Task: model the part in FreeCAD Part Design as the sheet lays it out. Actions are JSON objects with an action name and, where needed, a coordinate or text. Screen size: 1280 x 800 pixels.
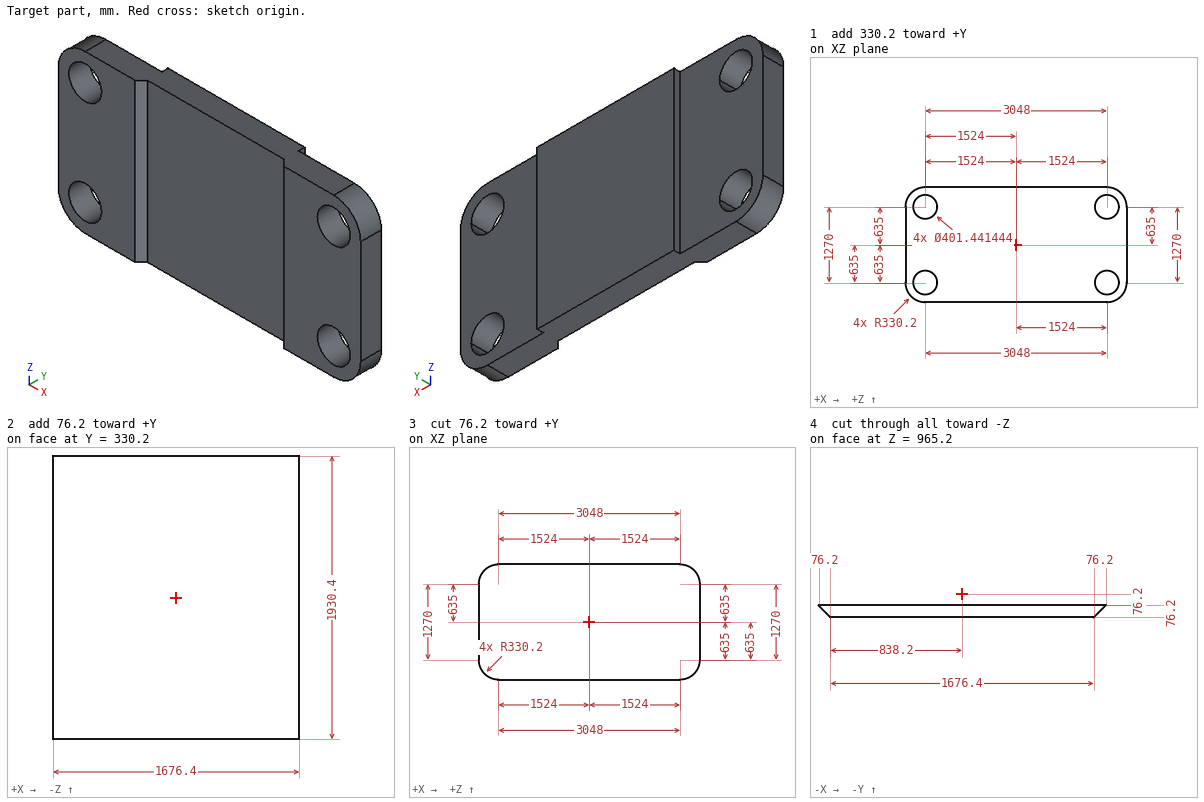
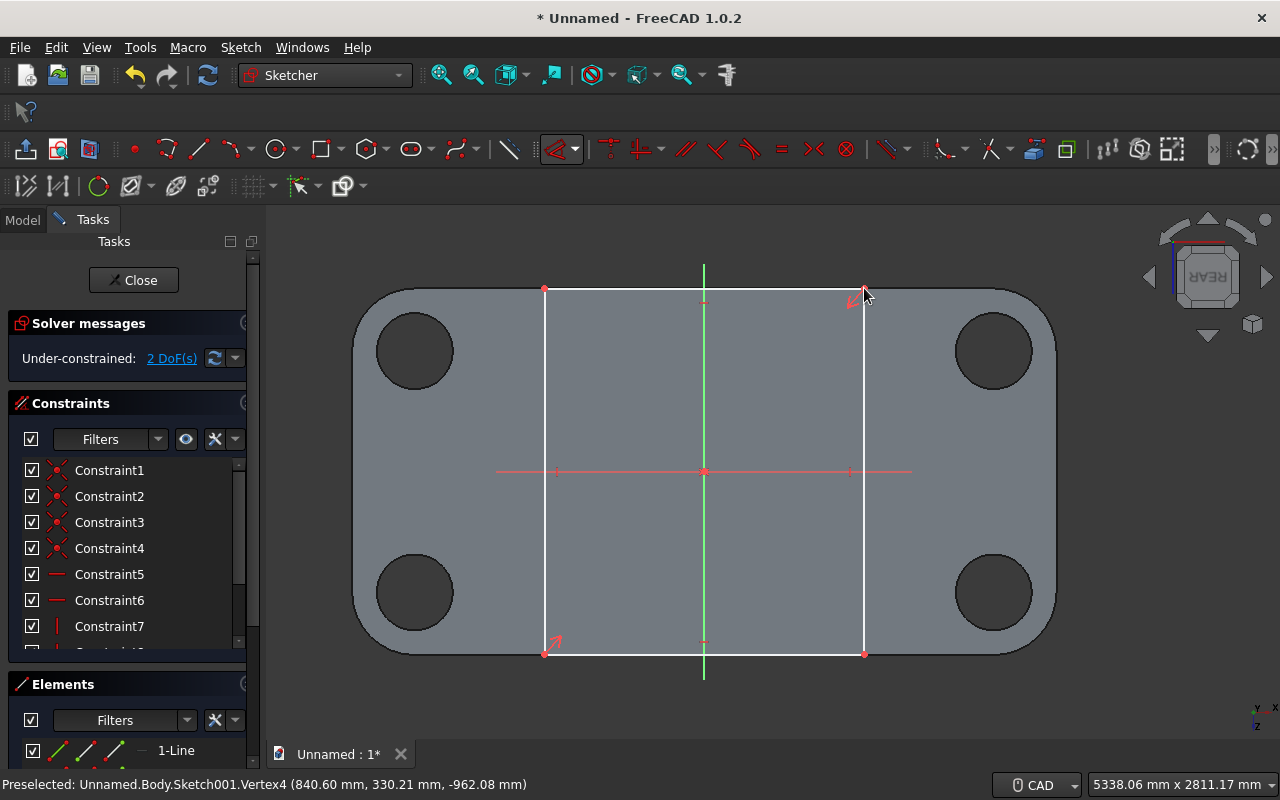
{"action": "left_click", "coordinate": [640, 655]}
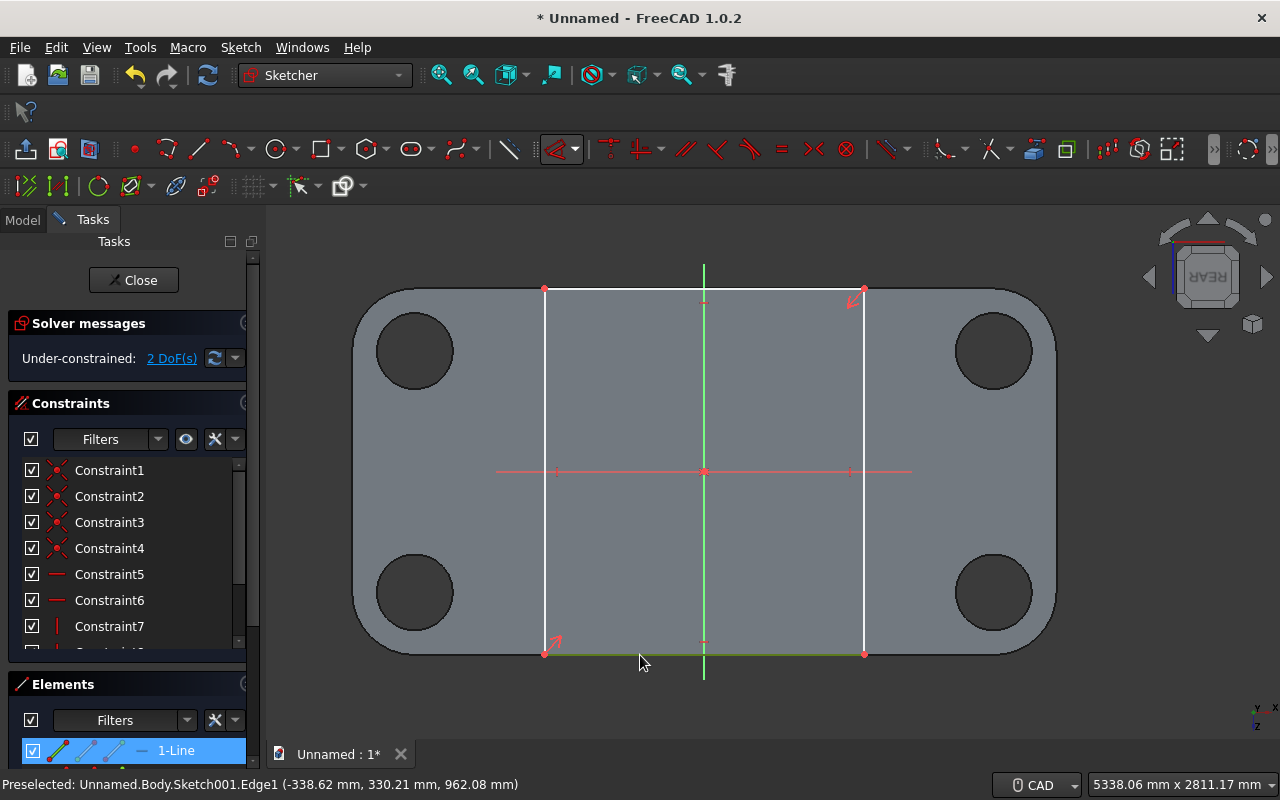
{"action": "key", "text": "l"}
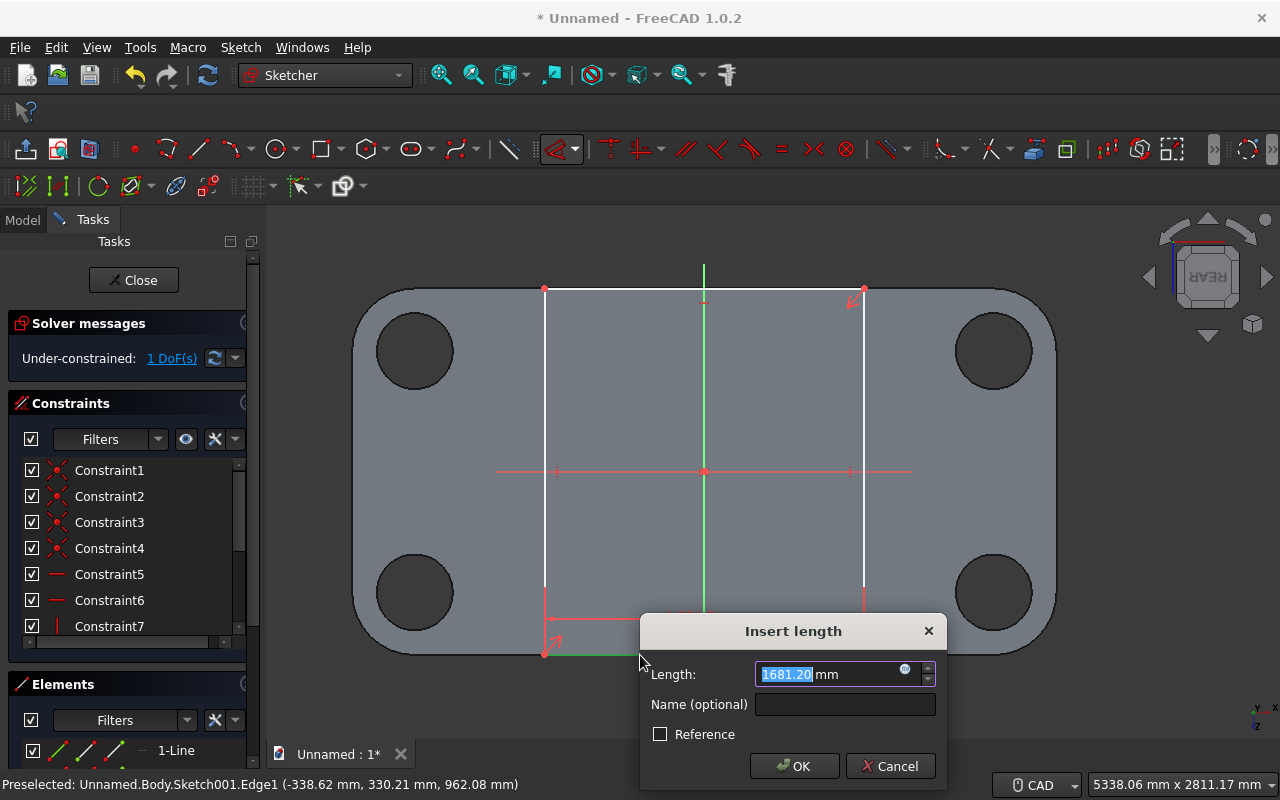
{"action": "type", "text": "1676.4"}
{"action": "key", "text": "Return"}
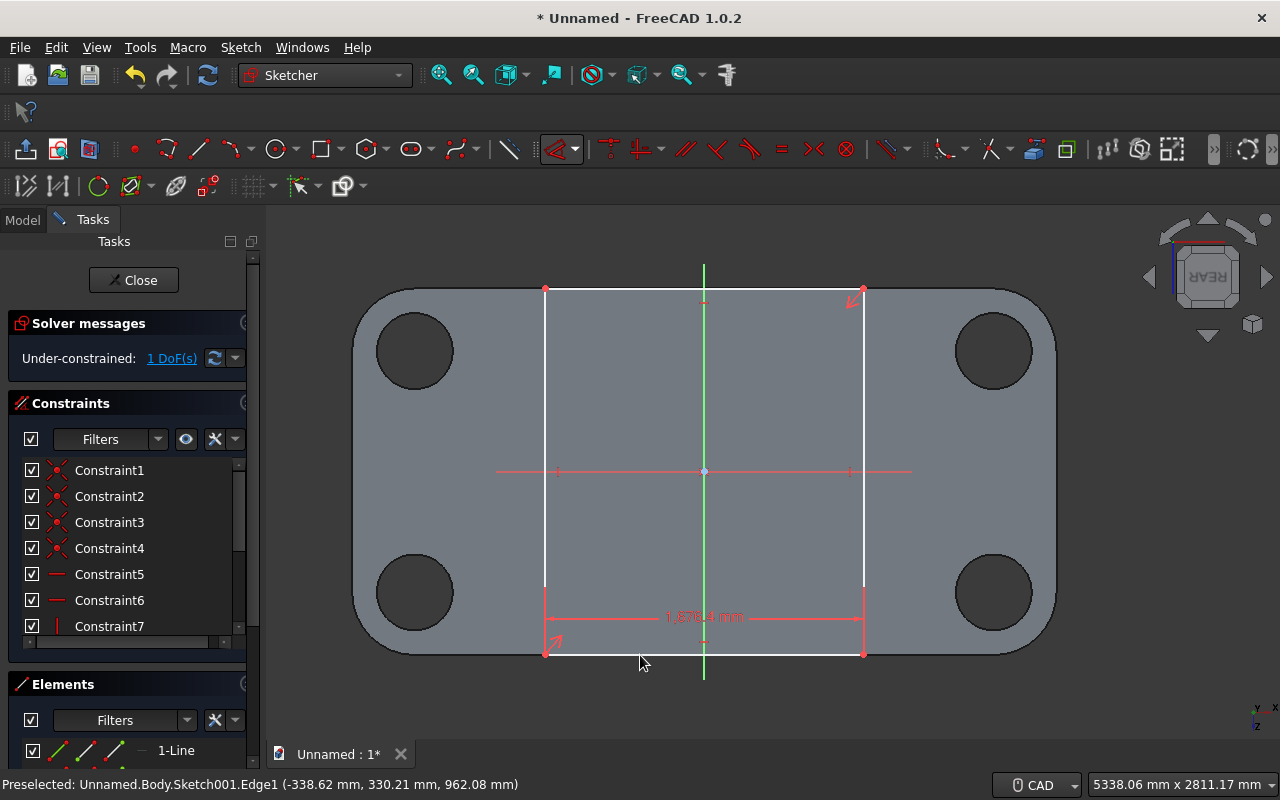
{"action": "left_click", "coordinate": [864, 545]}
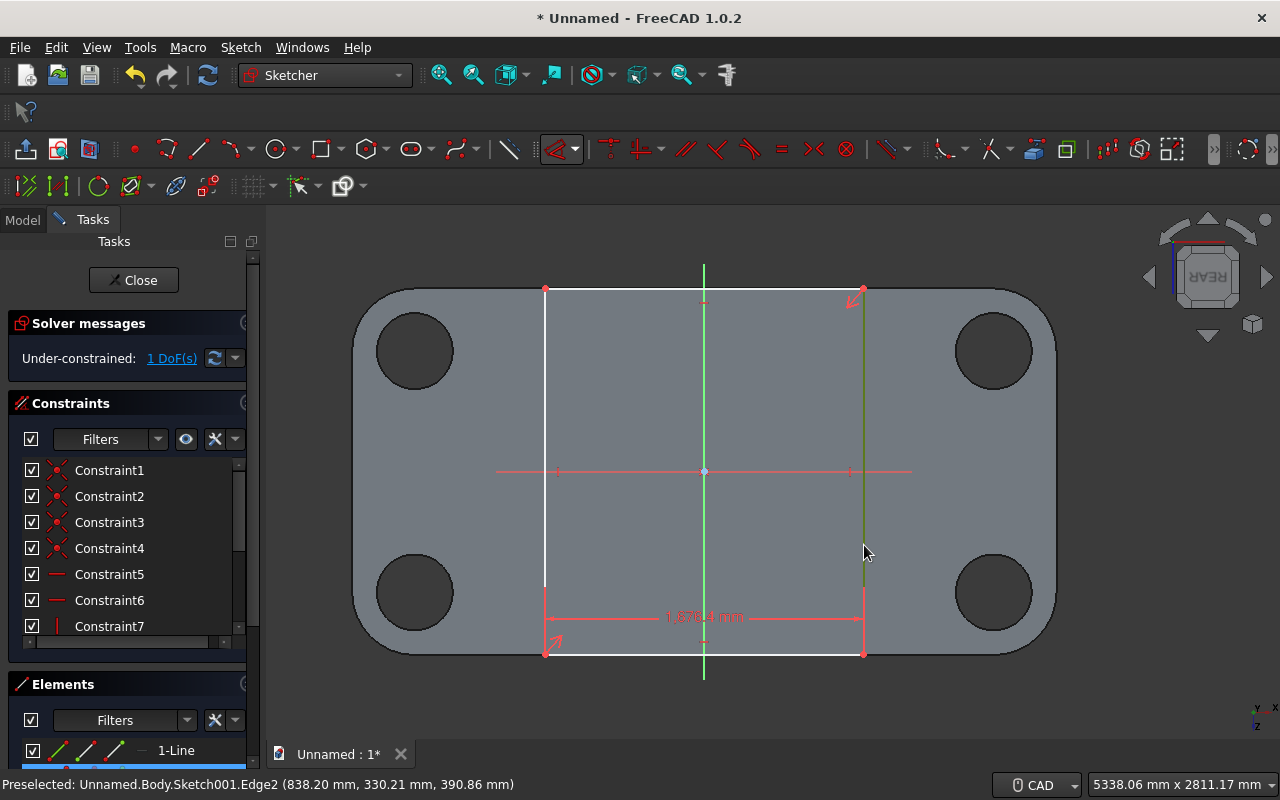
{"action": "key", "text": "i"}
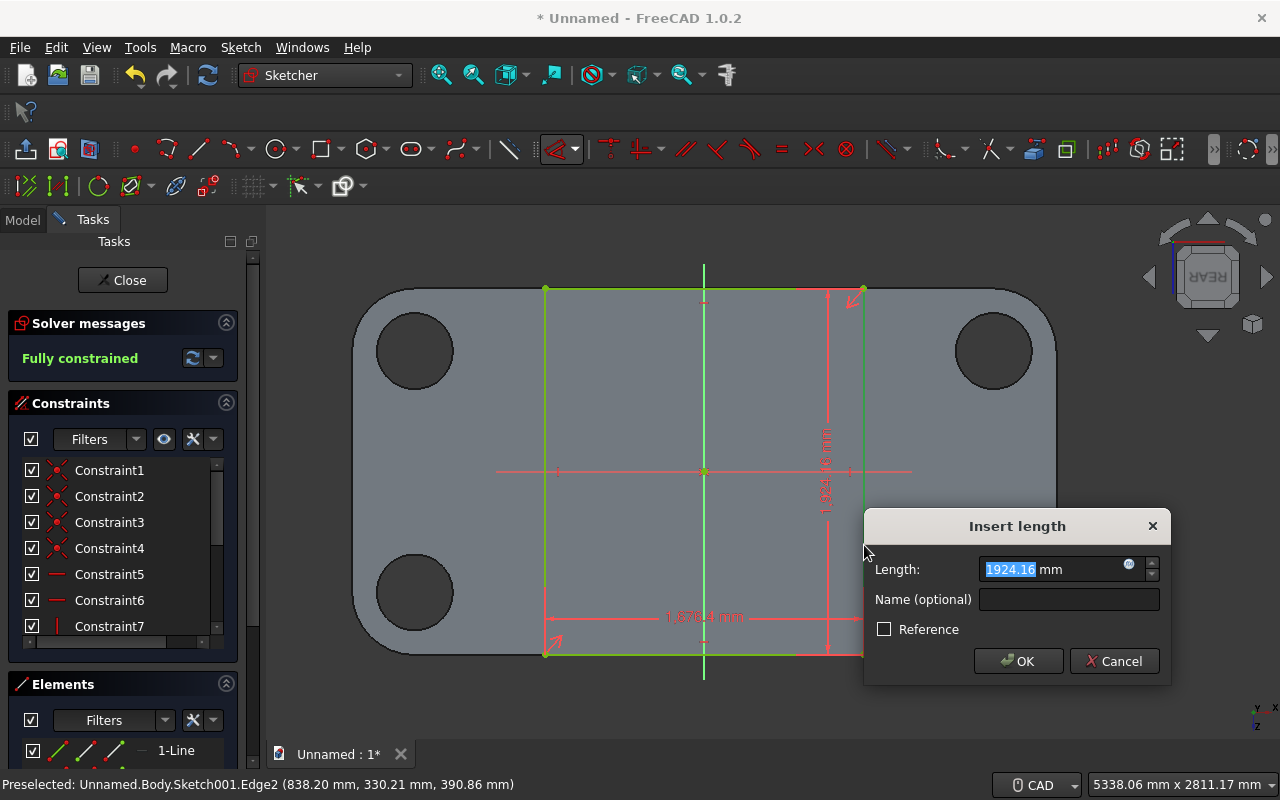
{"action": "type", "text": "1930.4"}
{"action": "key", "text": "Return"}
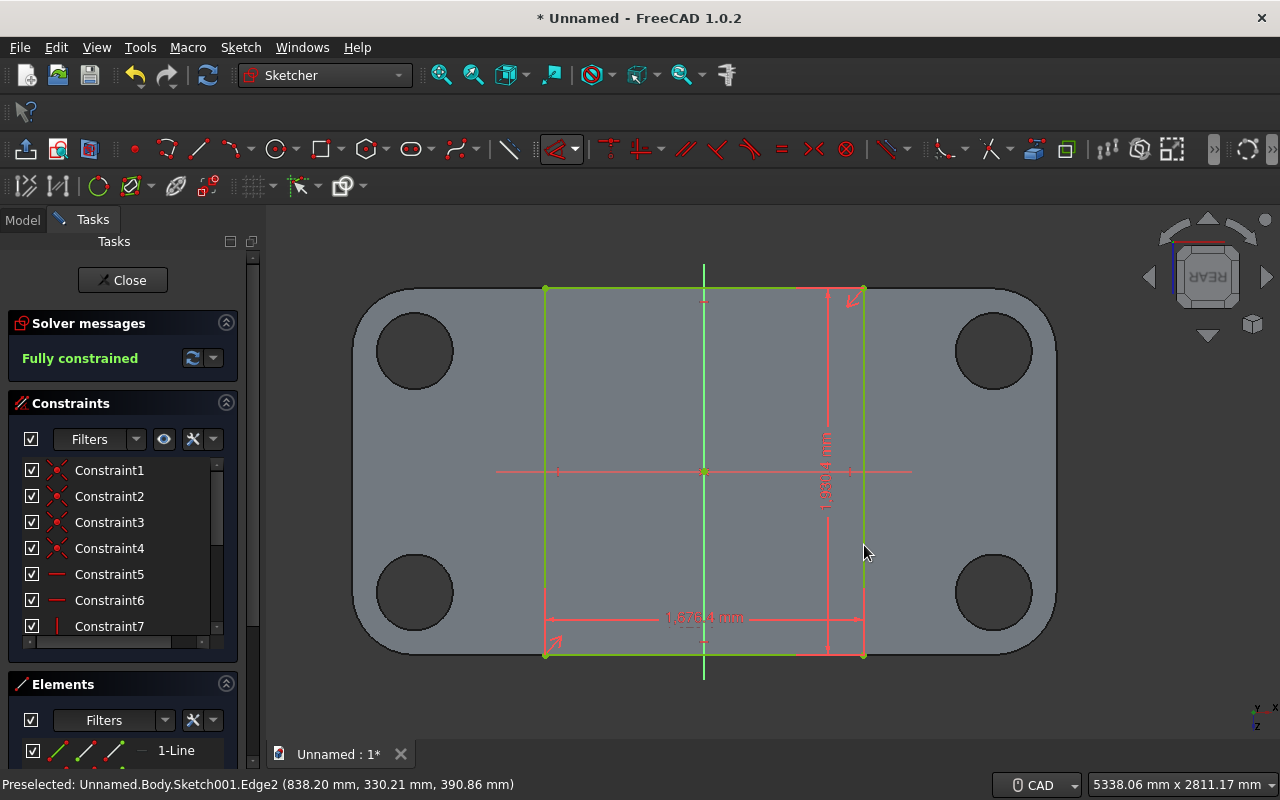
{"action": "left_click", "coordinate": [123, 280]}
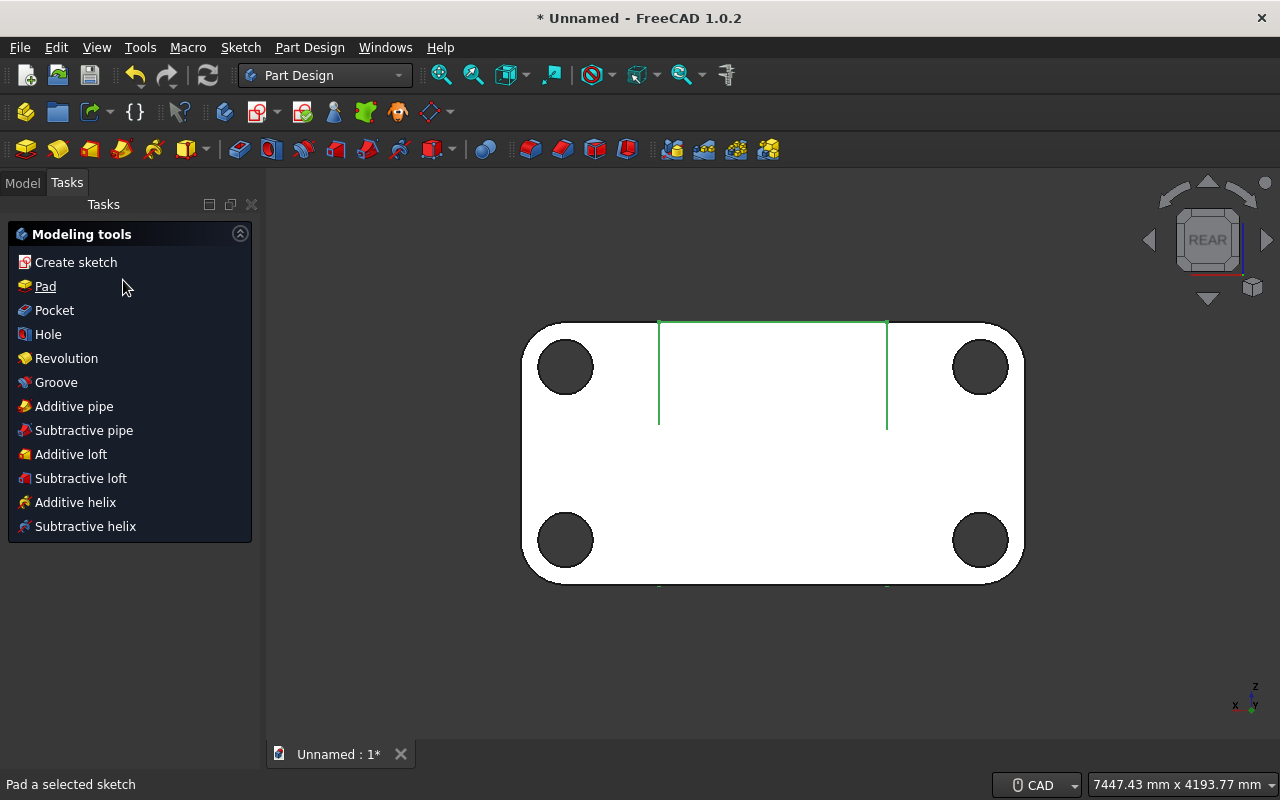
{"action": "left_click", "coordinate": [26, 150]}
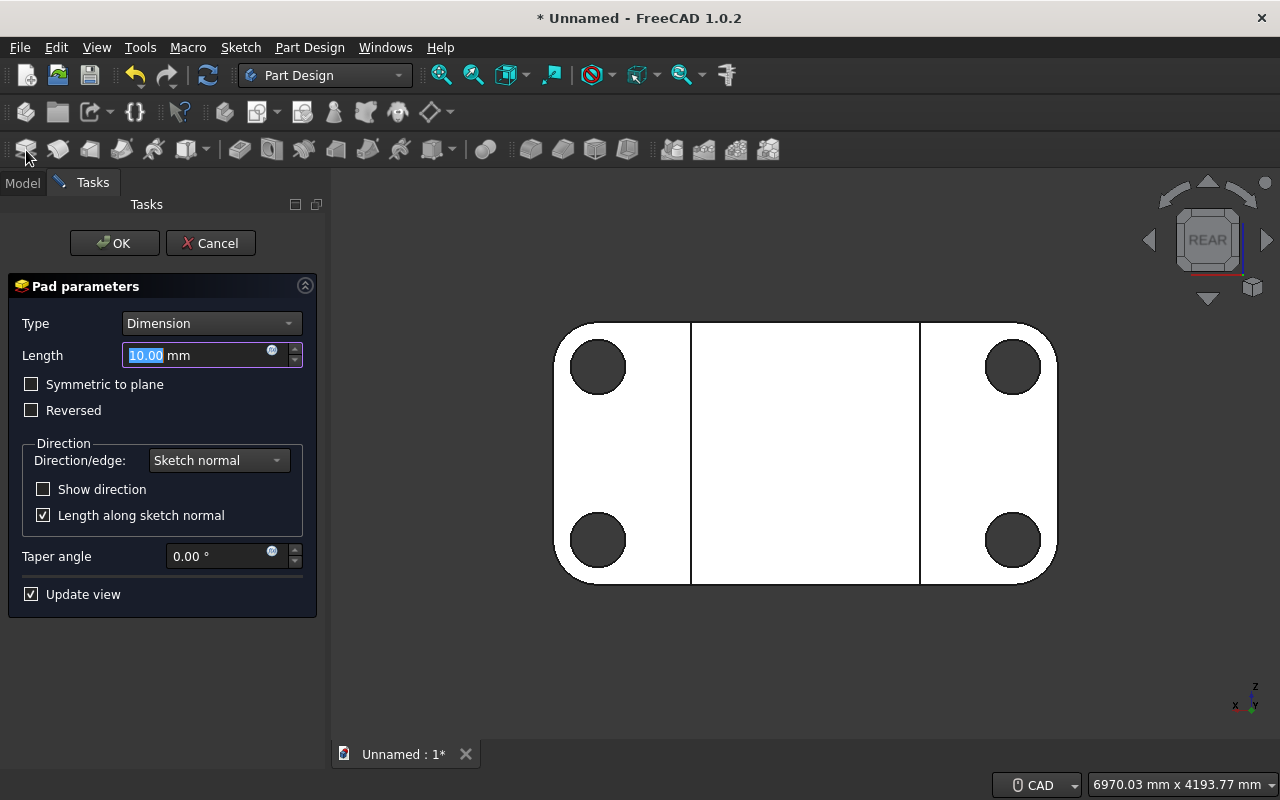
{"action": "type", "text": "76.2"}
{"action": "key", "text": "Tab"}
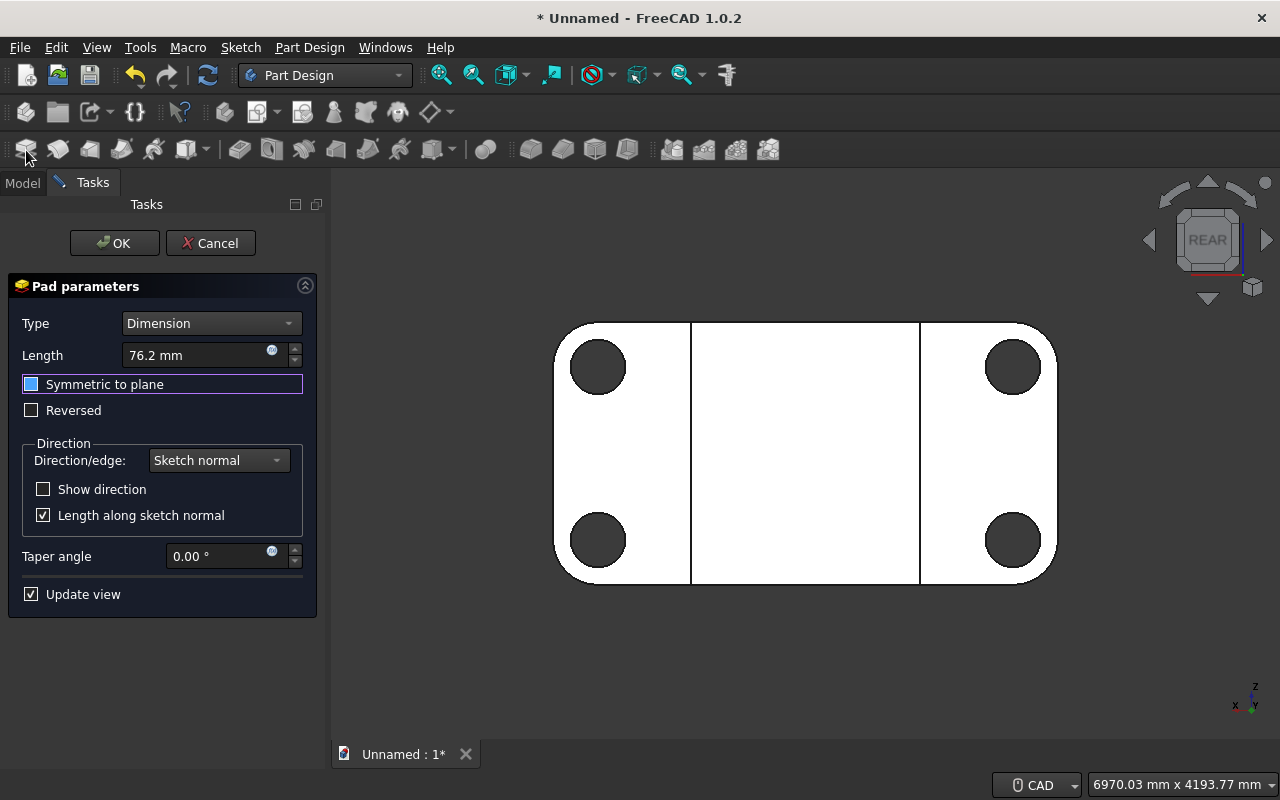
{"action": "left_click", "coordinate": [115, 243]}